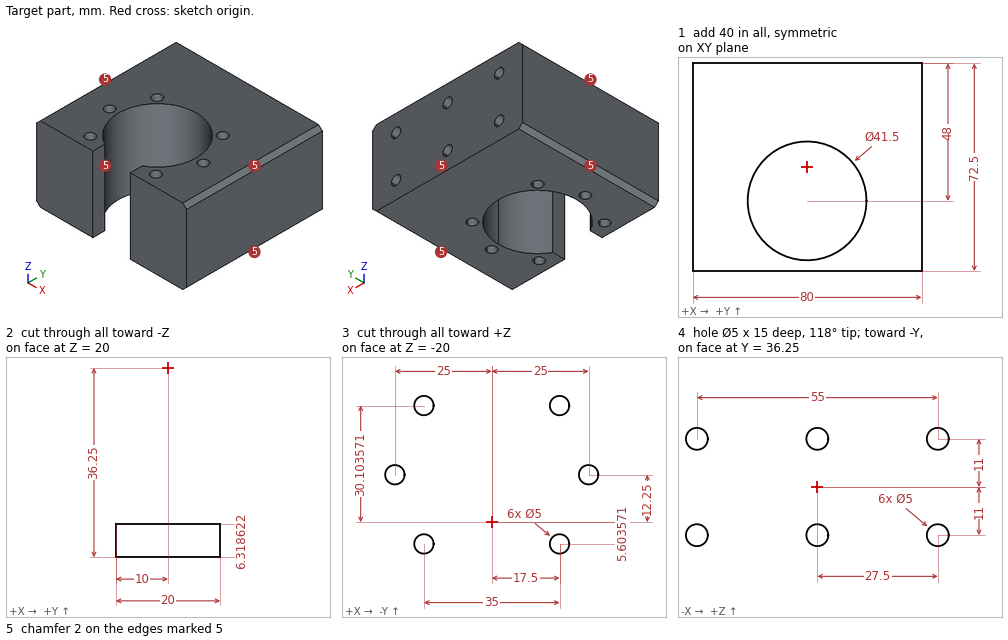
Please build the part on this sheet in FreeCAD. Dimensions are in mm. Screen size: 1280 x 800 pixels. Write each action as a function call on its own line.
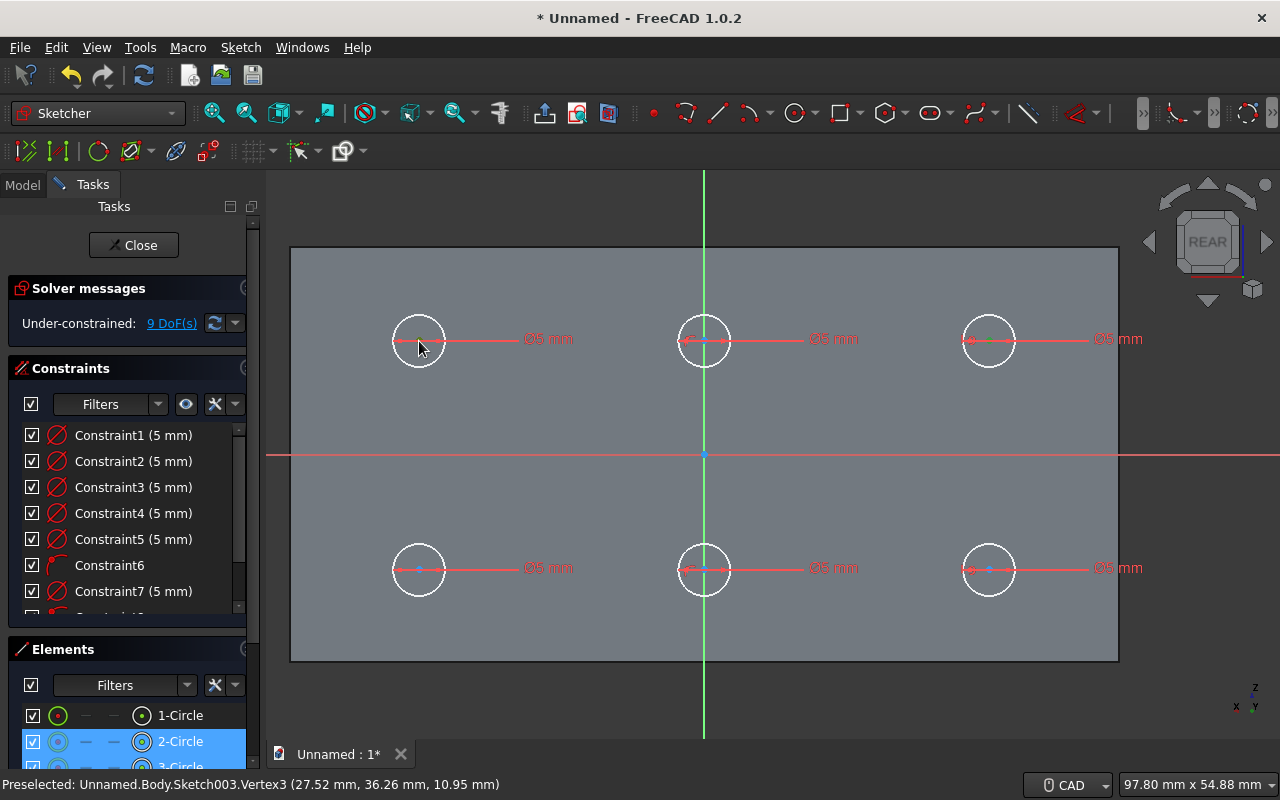
key(h)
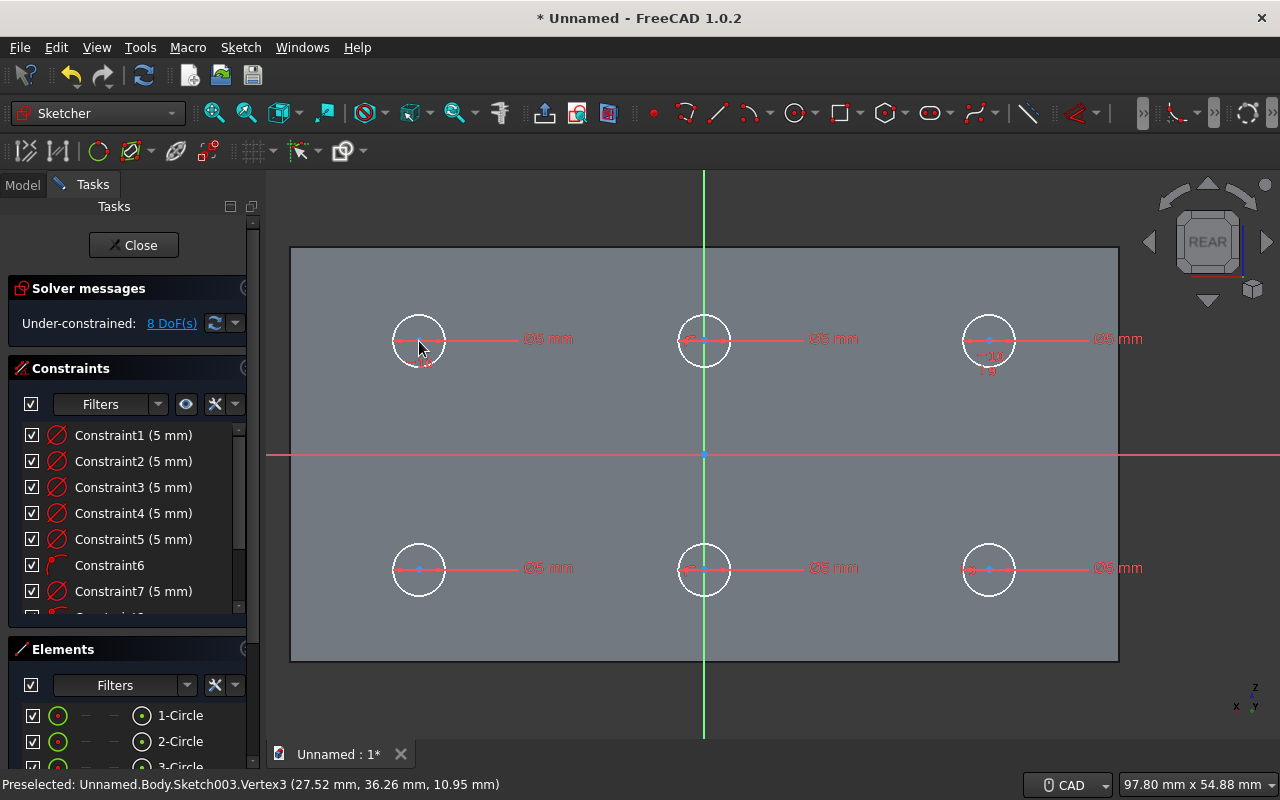
click(419, 341)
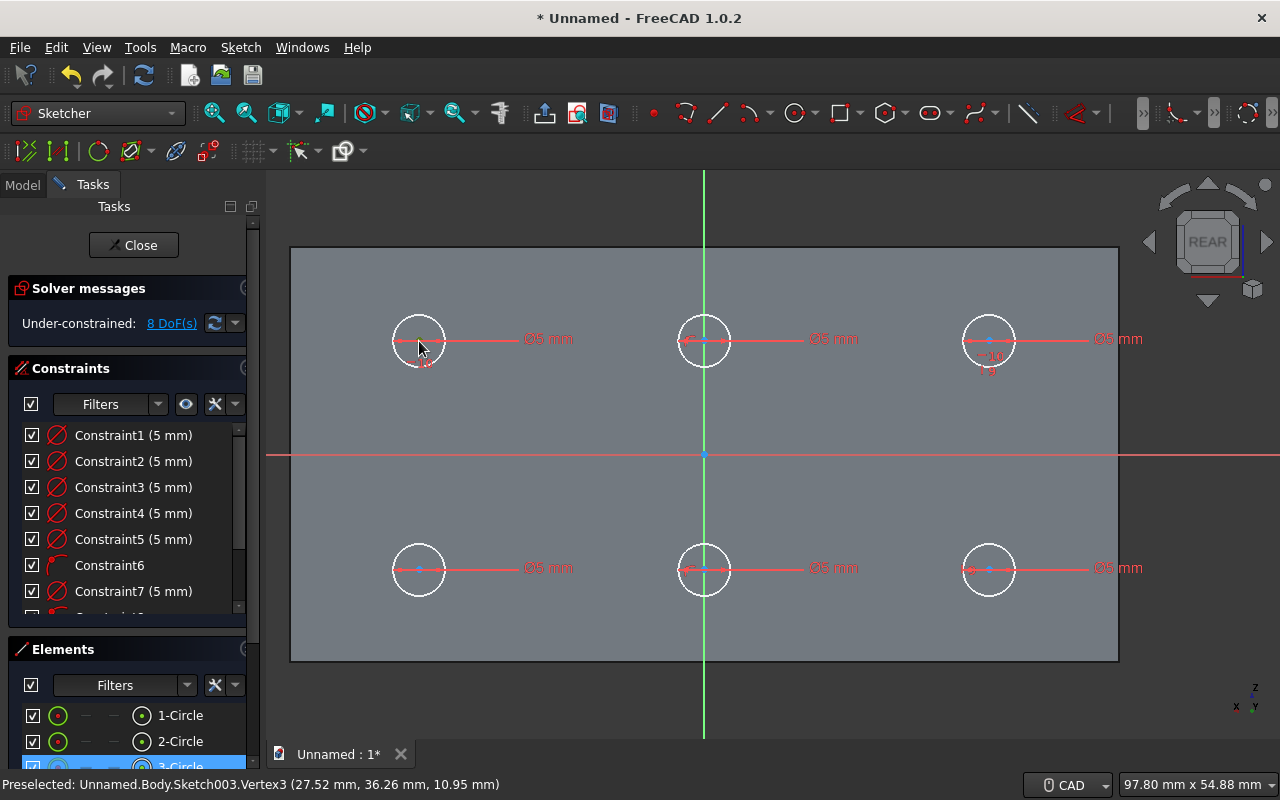
click(419, 570)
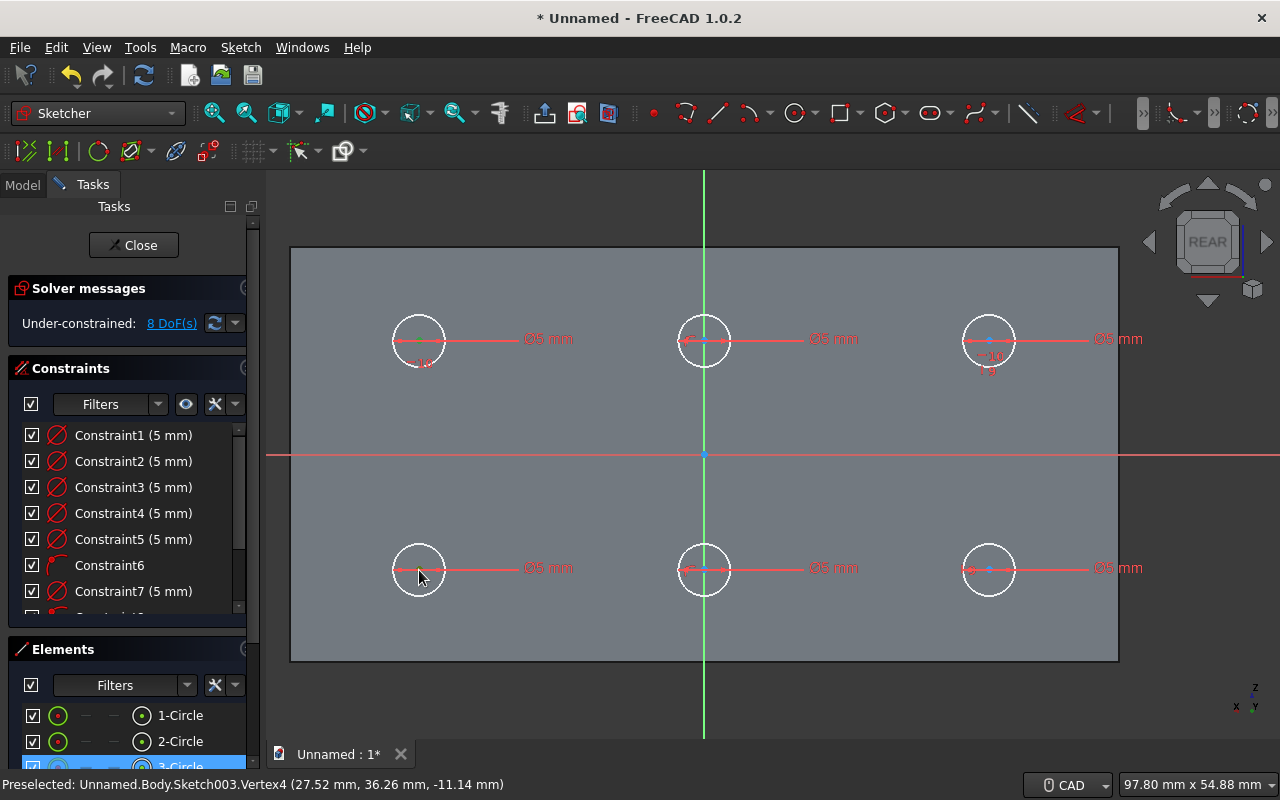
key(v)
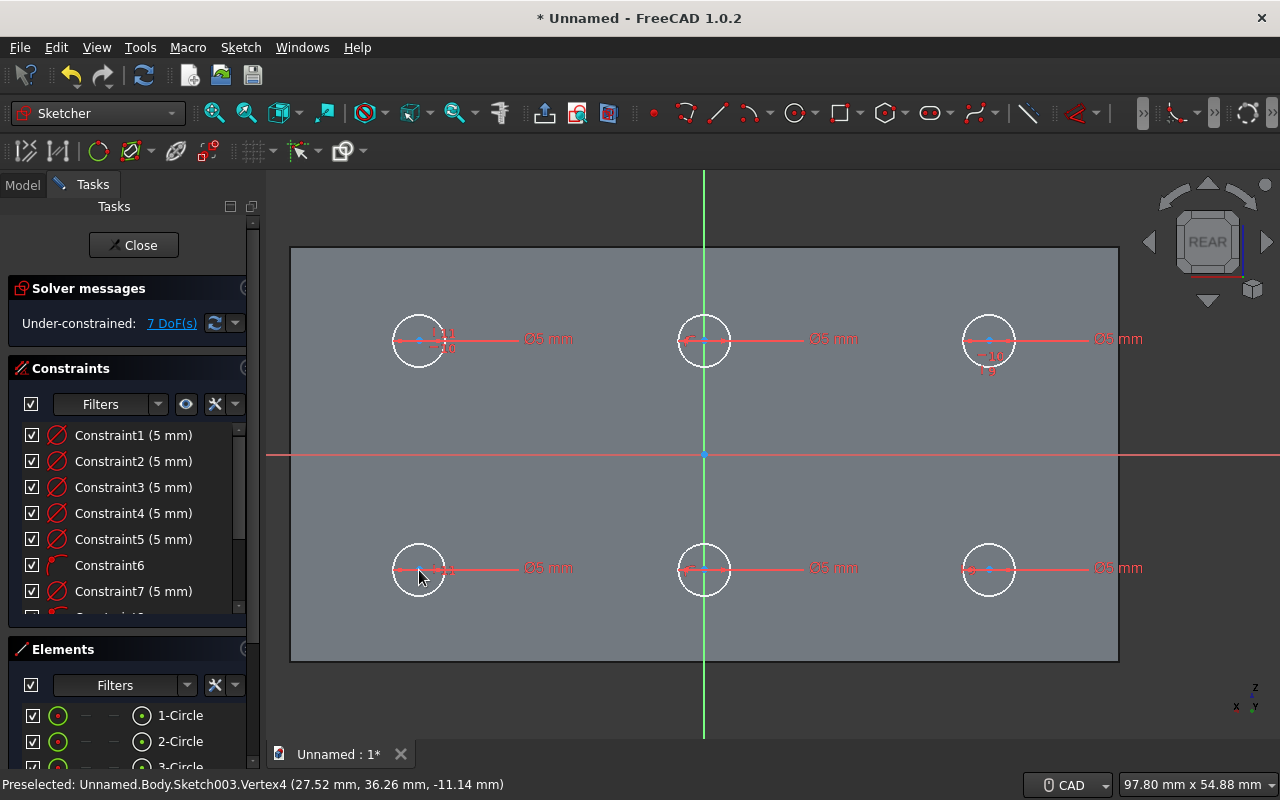
click(989, 570)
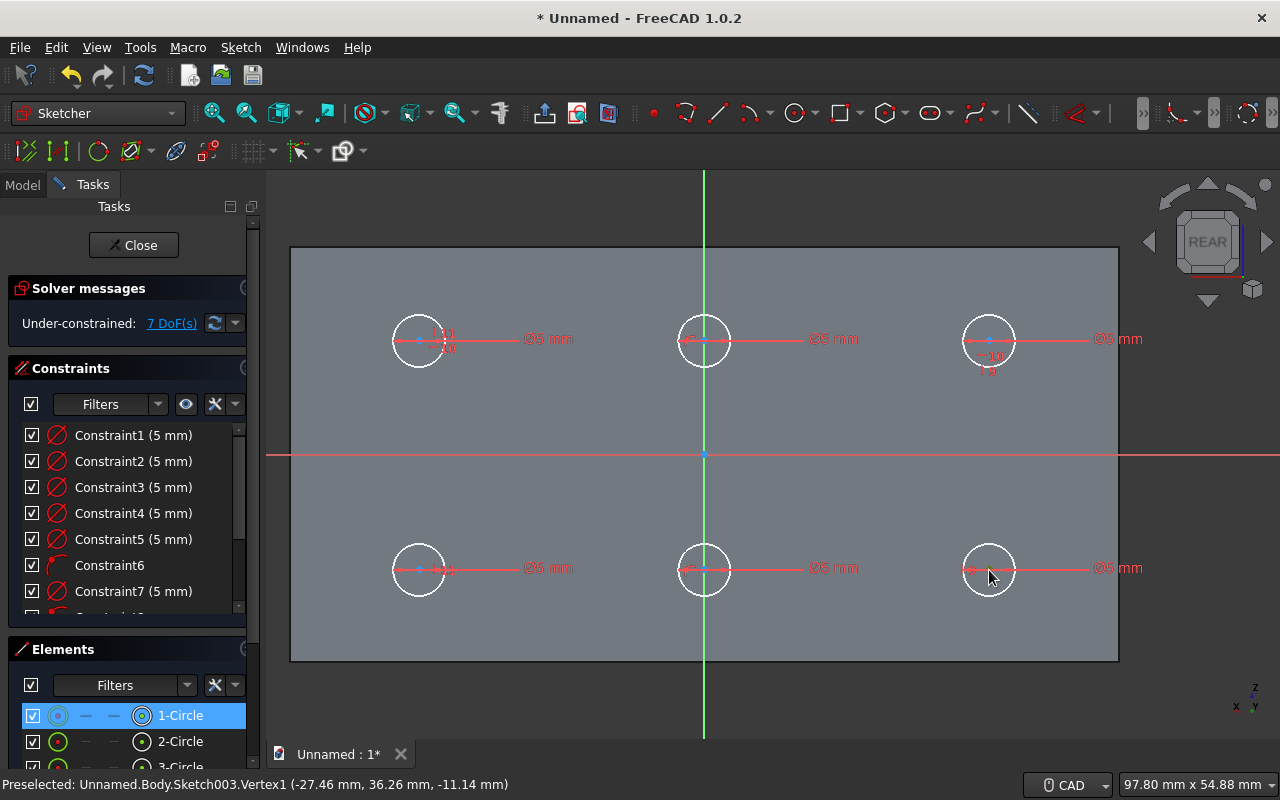
click(419, 570)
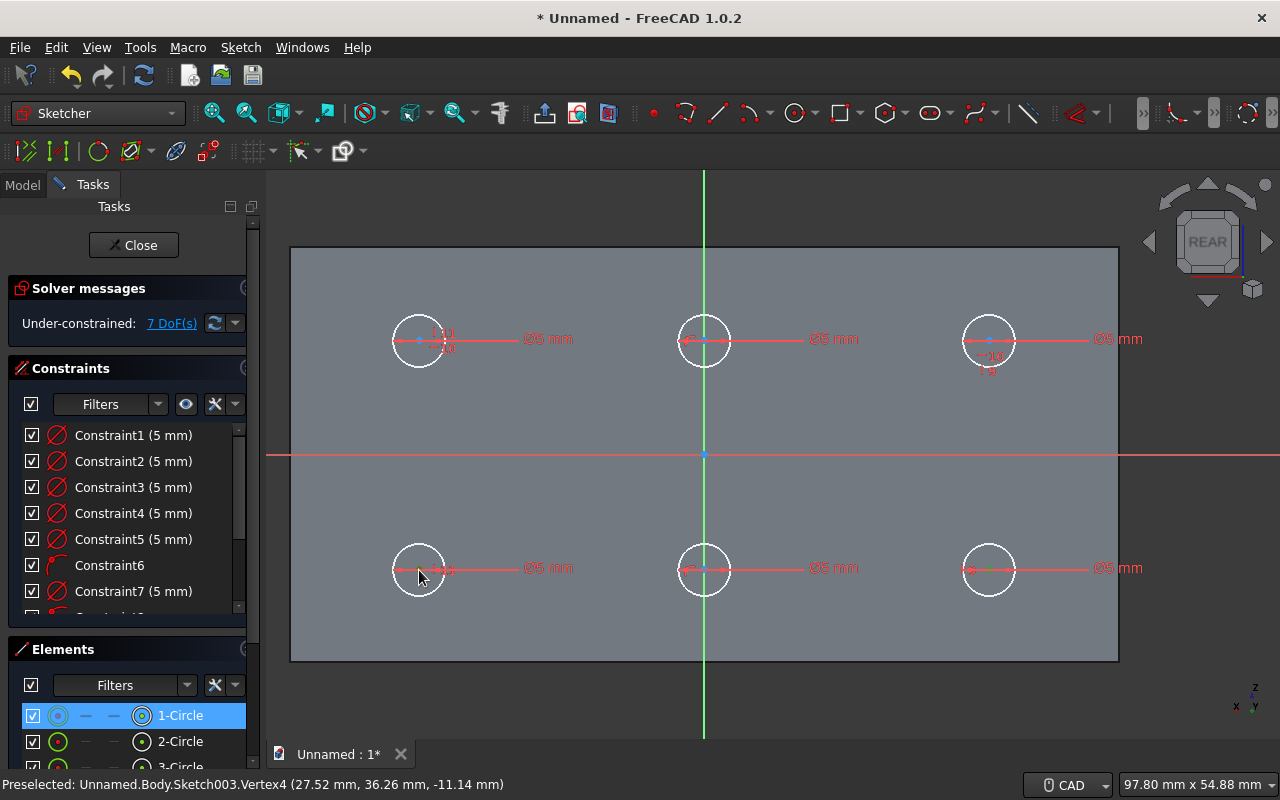
key(h)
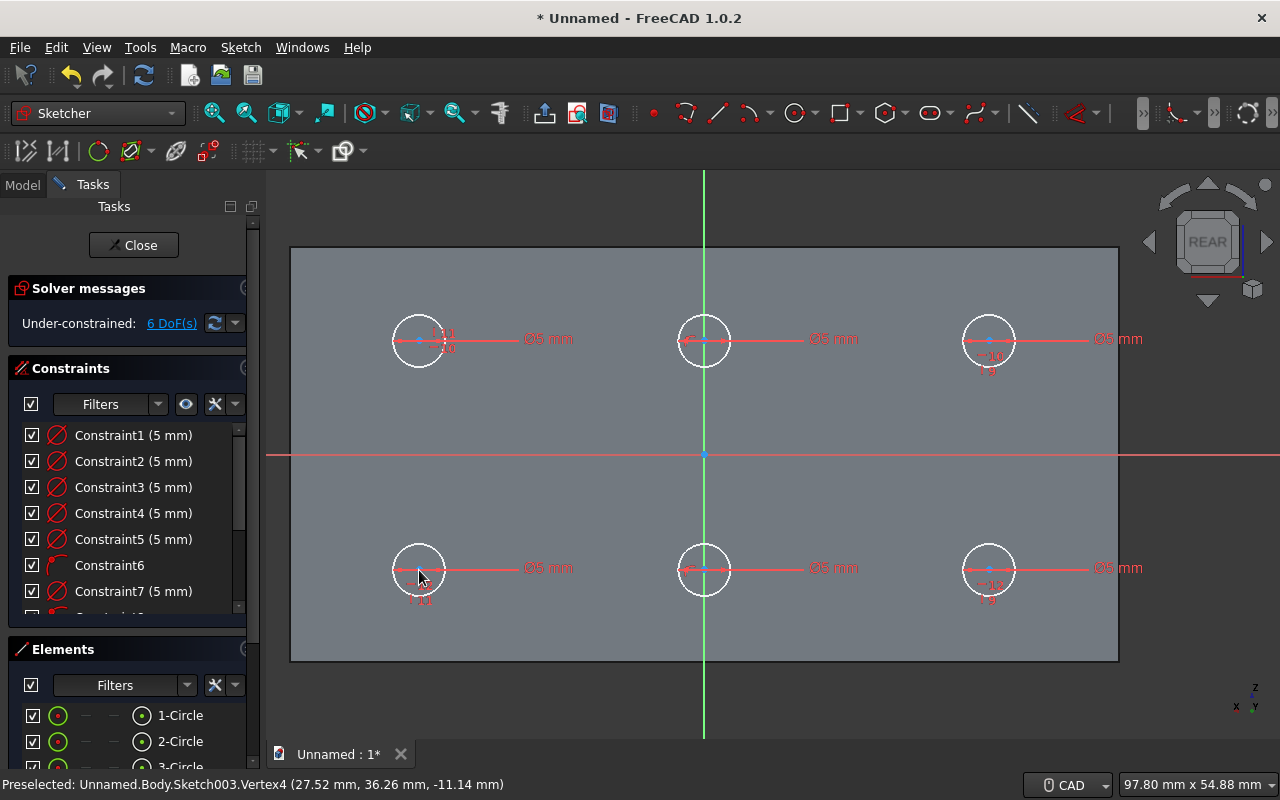
click(989, 570)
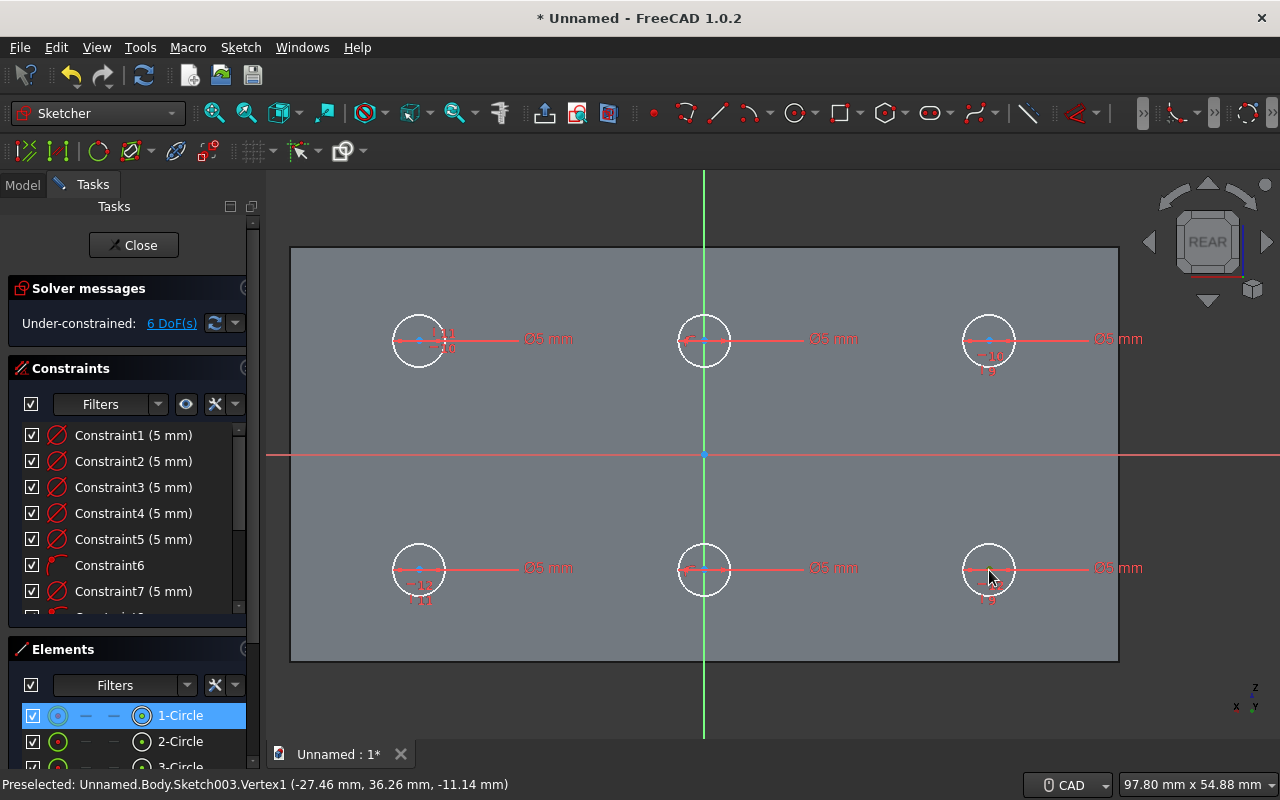
click(704, 570)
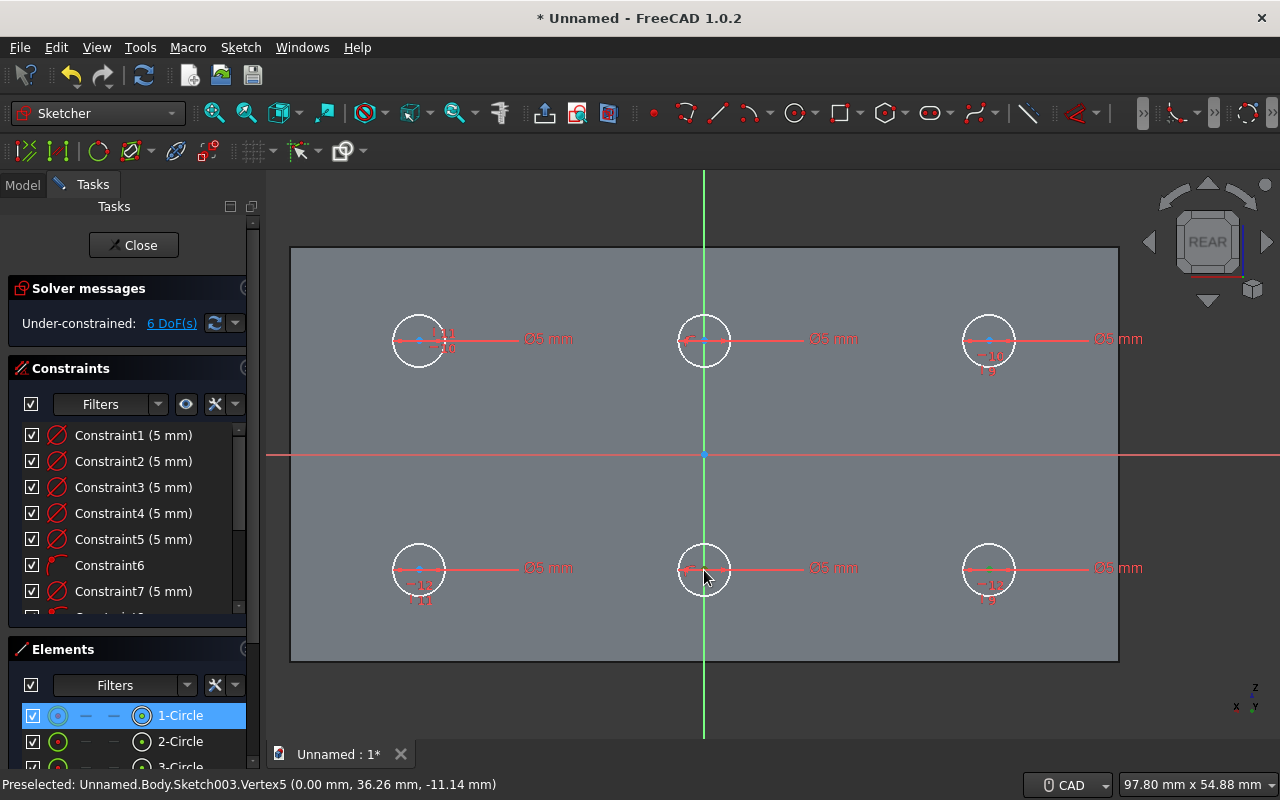
key(h)